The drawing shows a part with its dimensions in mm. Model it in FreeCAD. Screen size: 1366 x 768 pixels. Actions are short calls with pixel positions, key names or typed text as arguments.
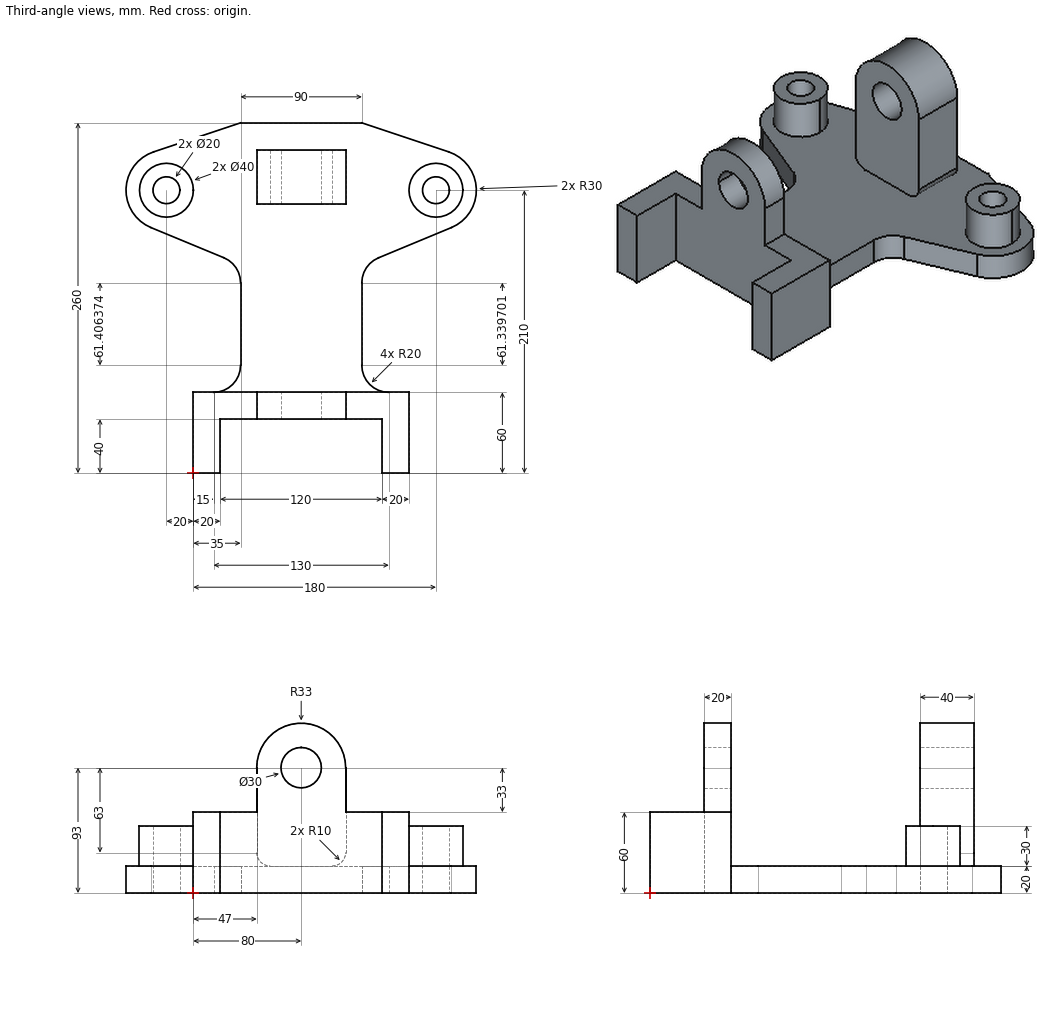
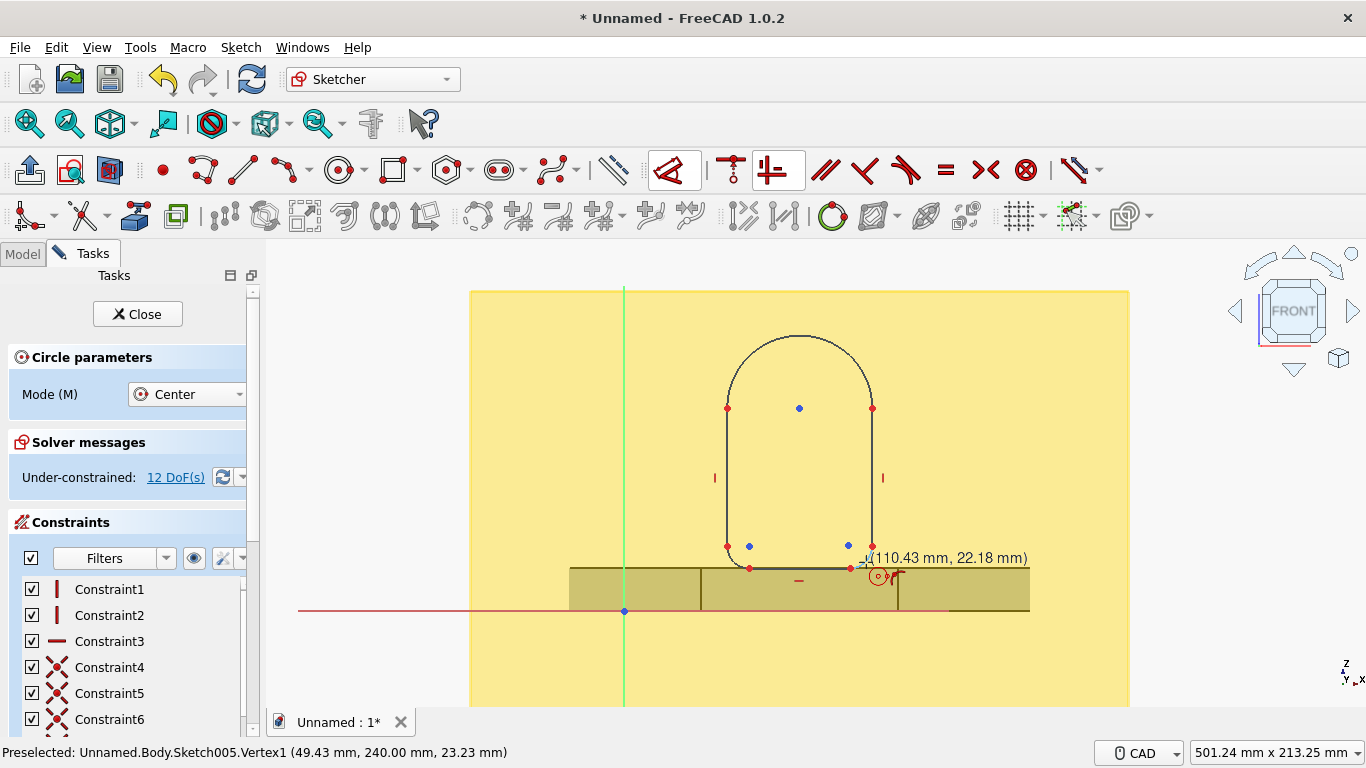
click(800, 407)
click(823, 384)
key(Escape)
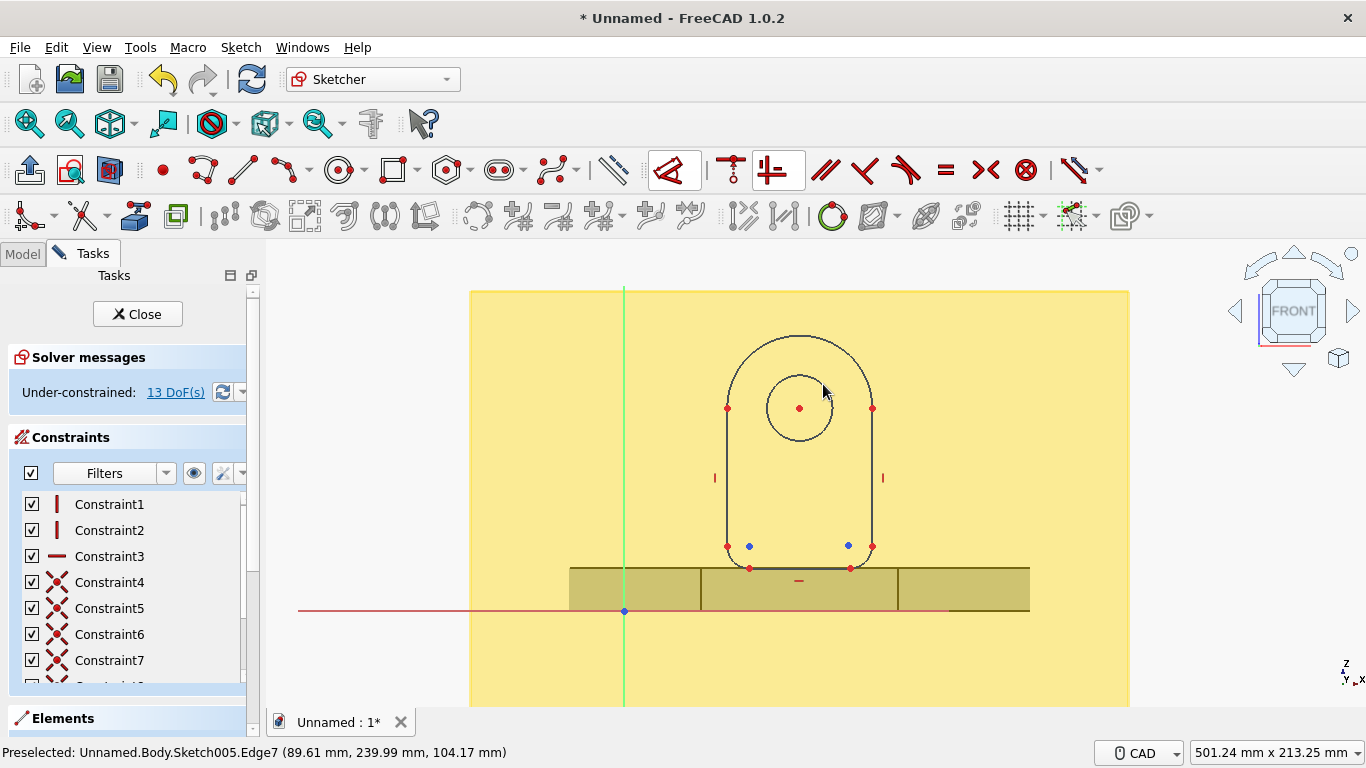
click(727, 505)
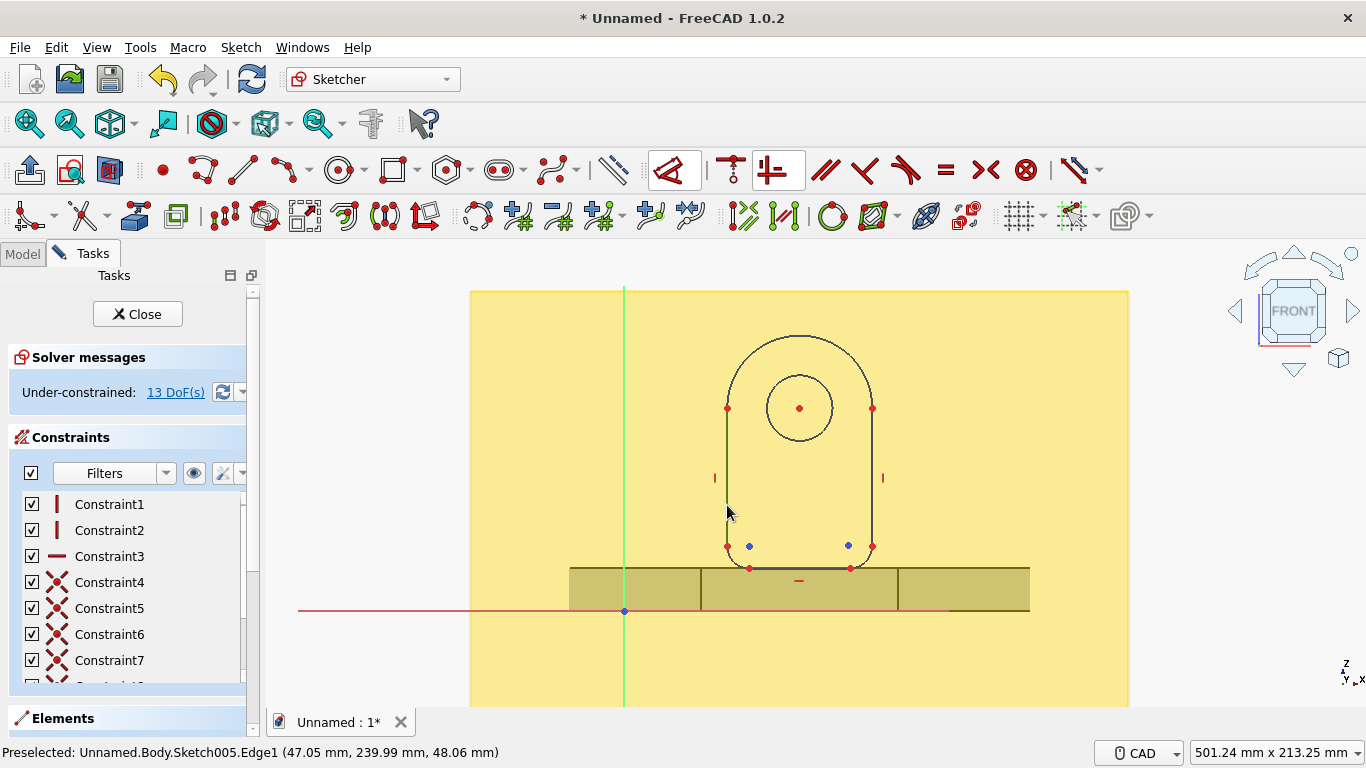
click(843, 350)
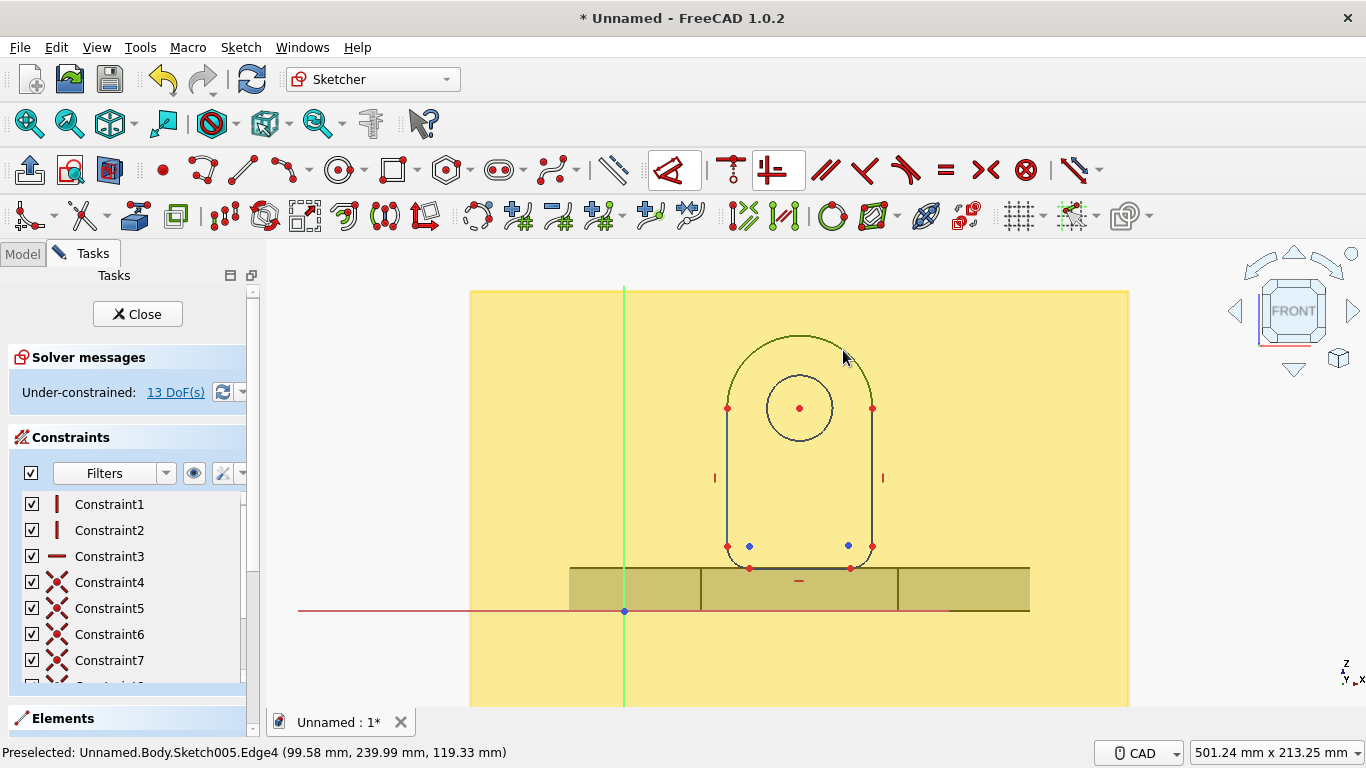
click(906, 170)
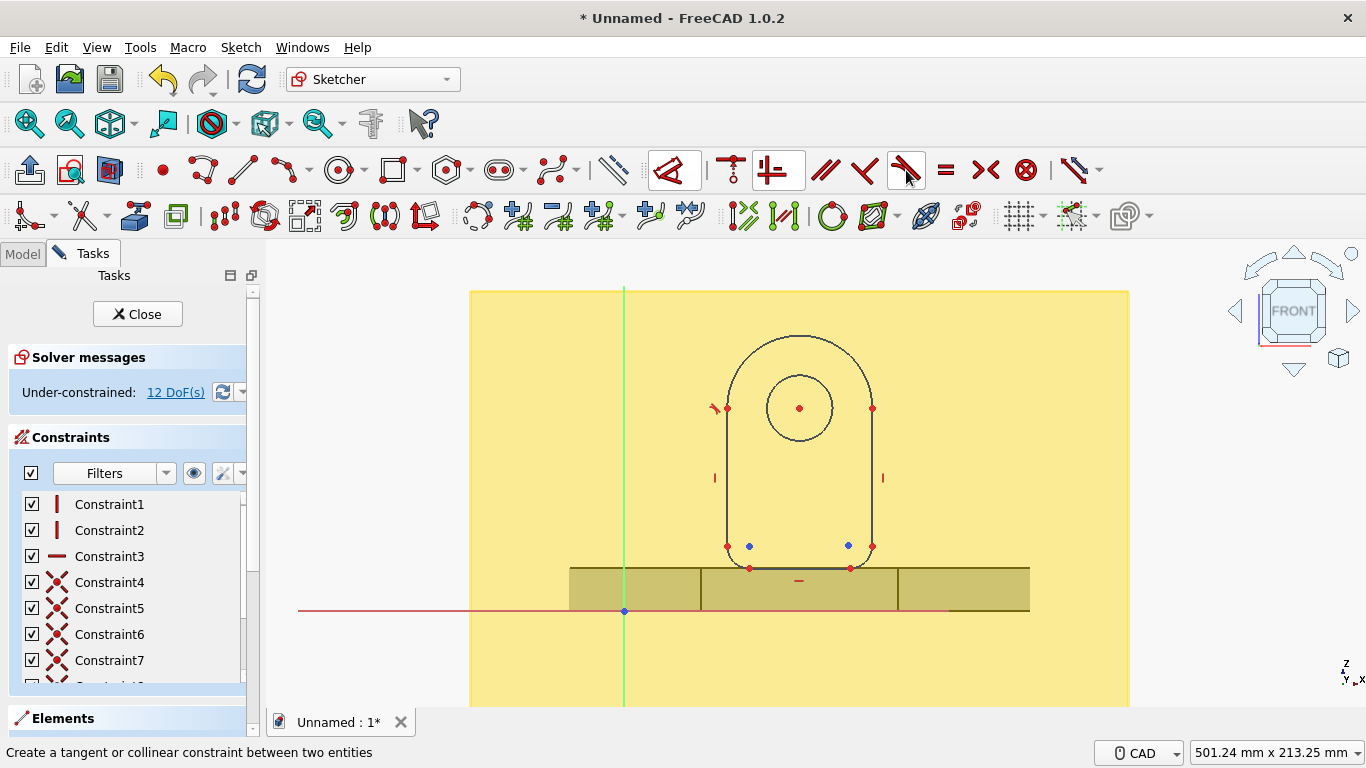
click(727, 505)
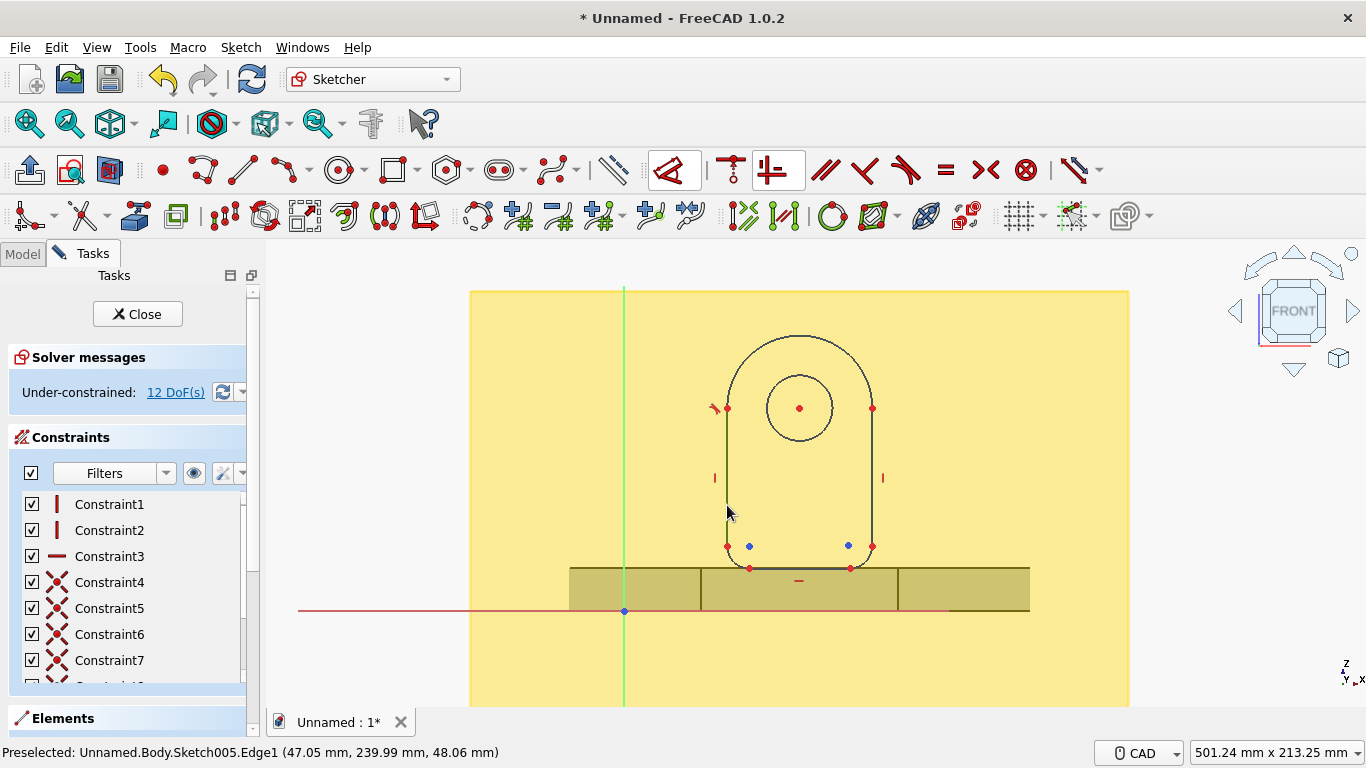
scroll(730, 557, up, 2)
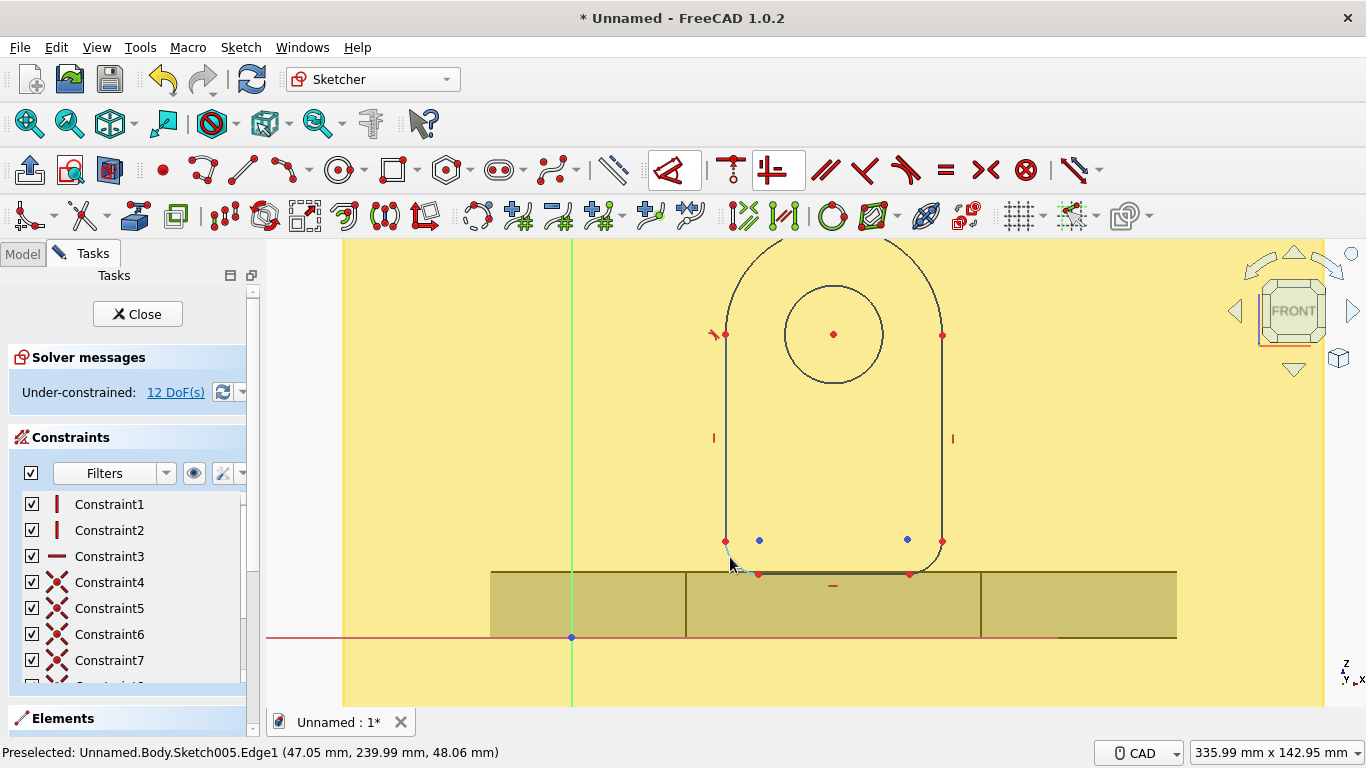
click(730, 556)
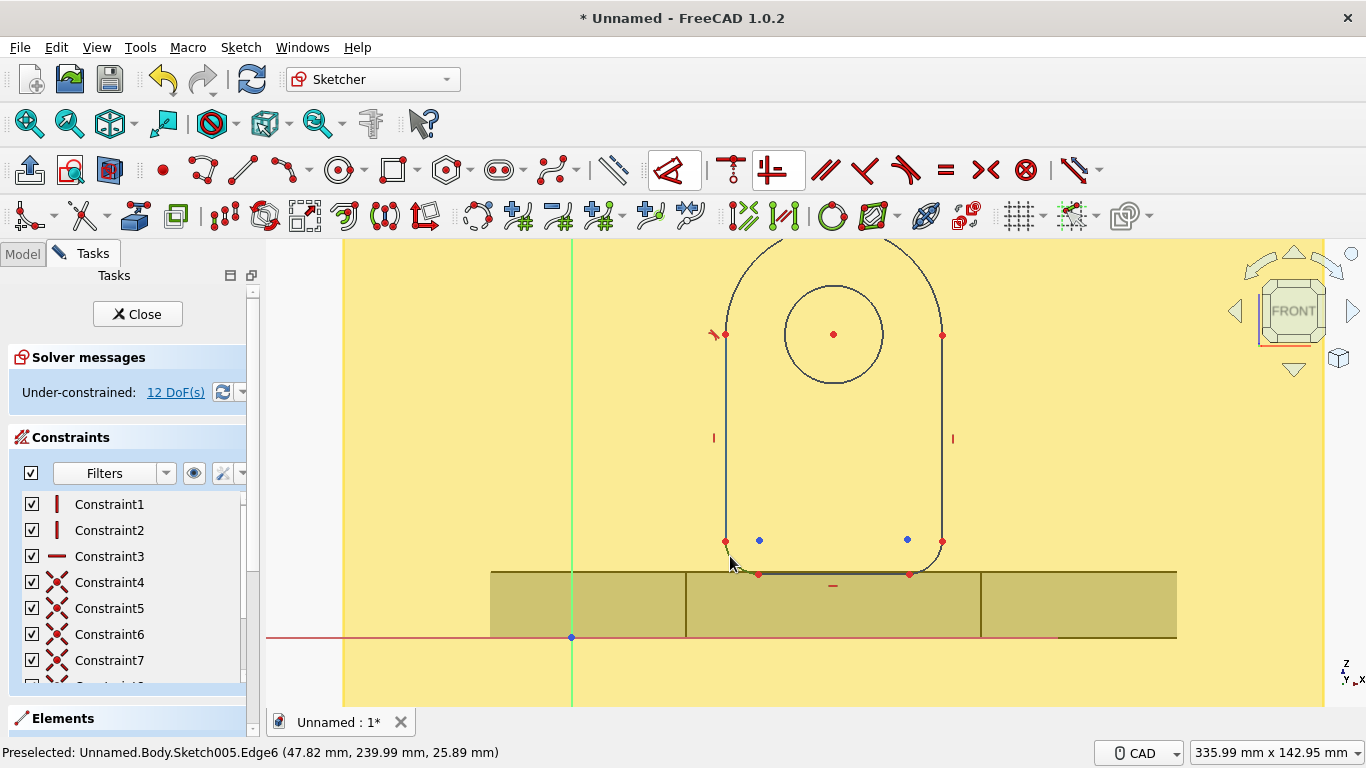
click(906, 170)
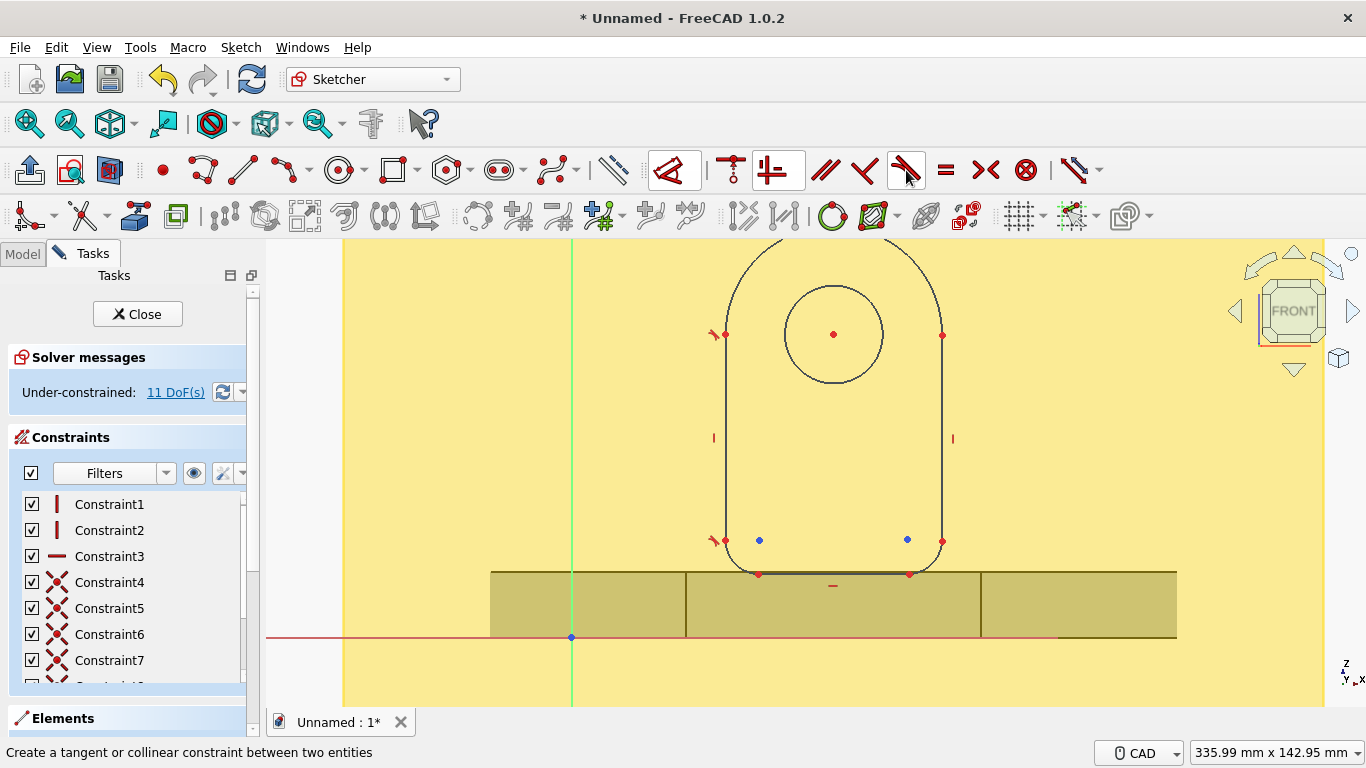
click(942, 397)